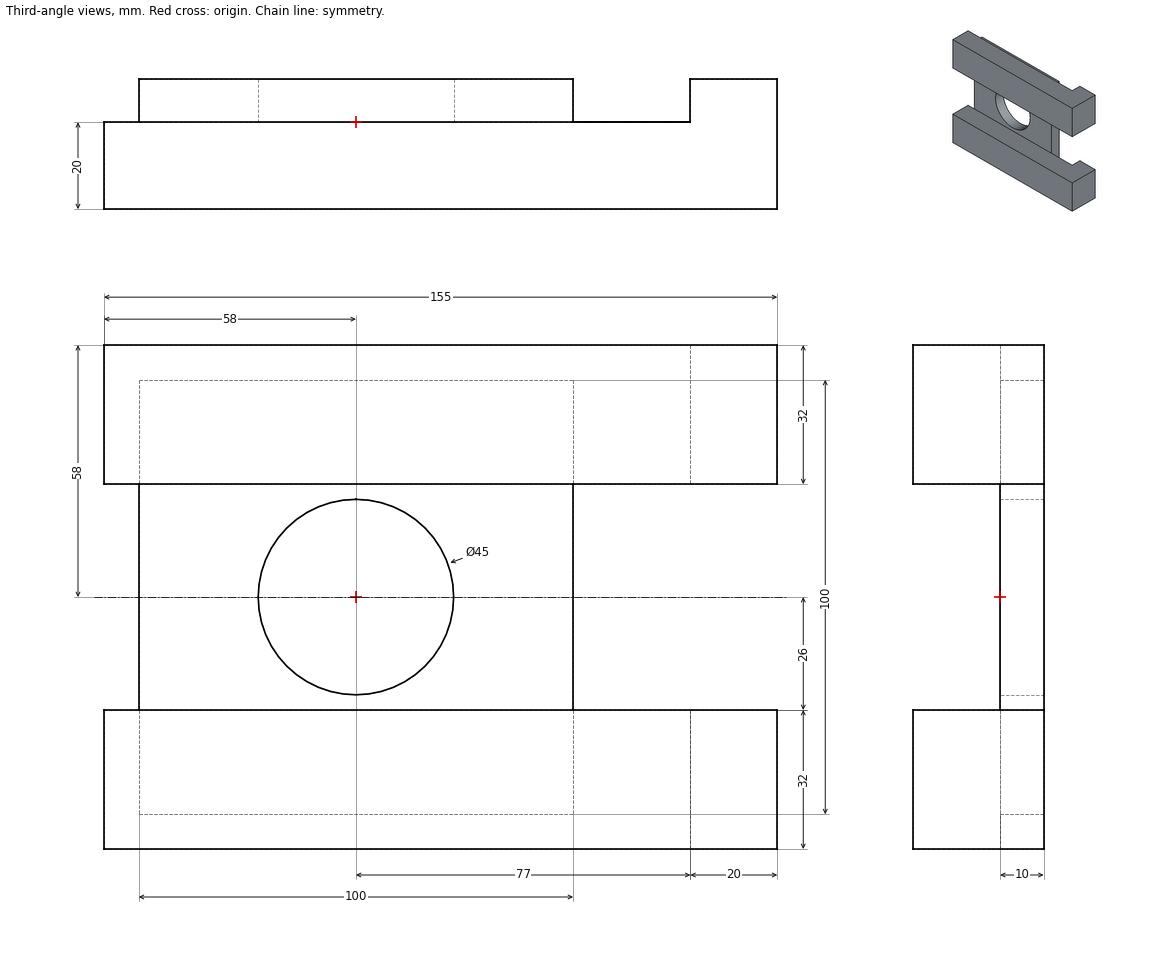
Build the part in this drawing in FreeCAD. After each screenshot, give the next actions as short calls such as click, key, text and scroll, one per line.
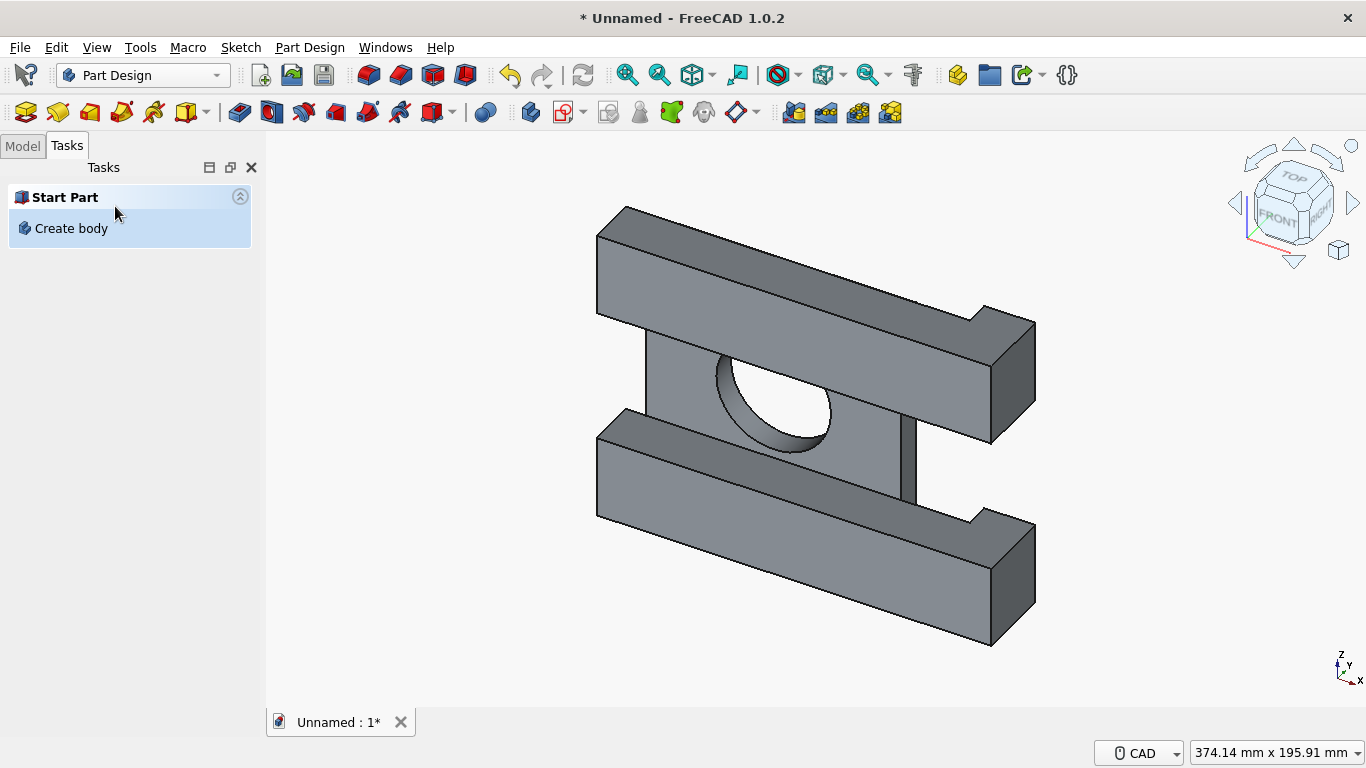
key(0)